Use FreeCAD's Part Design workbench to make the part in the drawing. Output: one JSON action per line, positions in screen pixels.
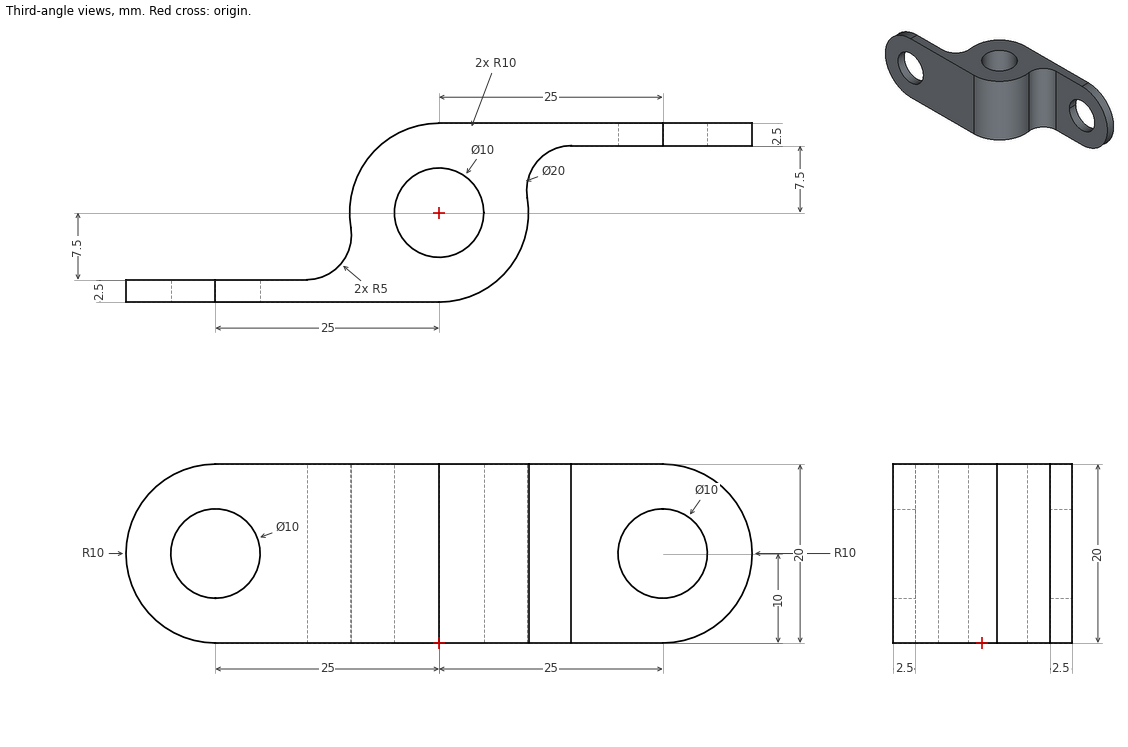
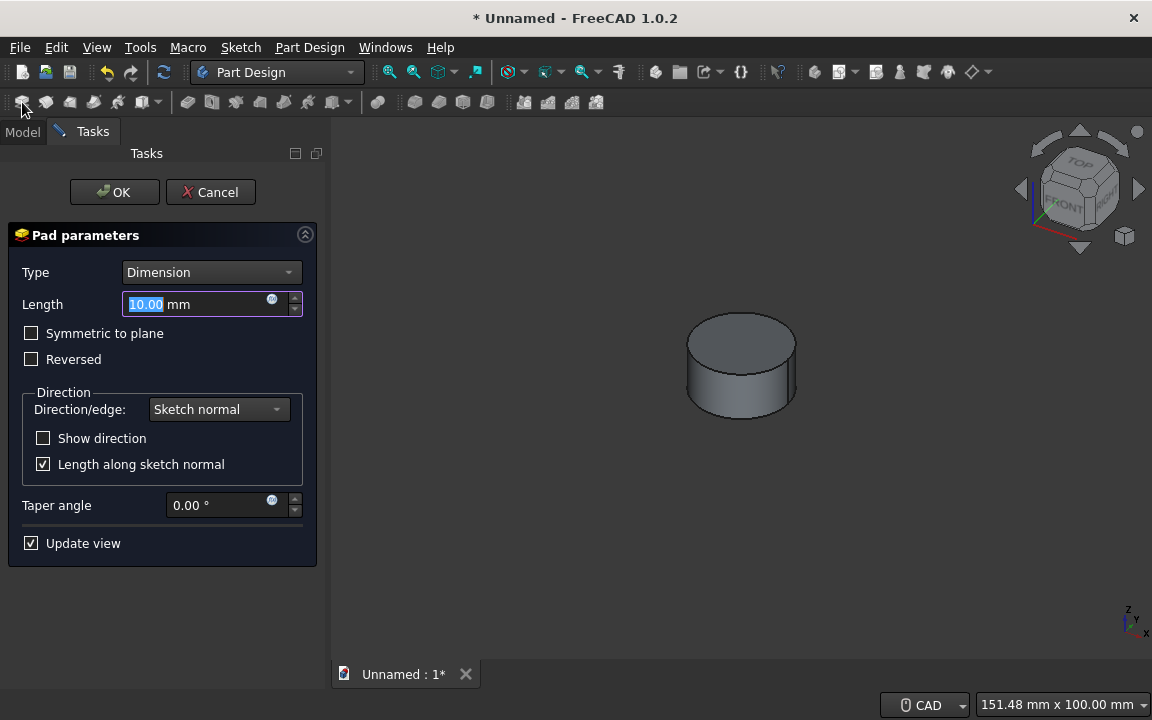
{"action": "type", "text": "20"}
{"action": "key", "text": "Tab"}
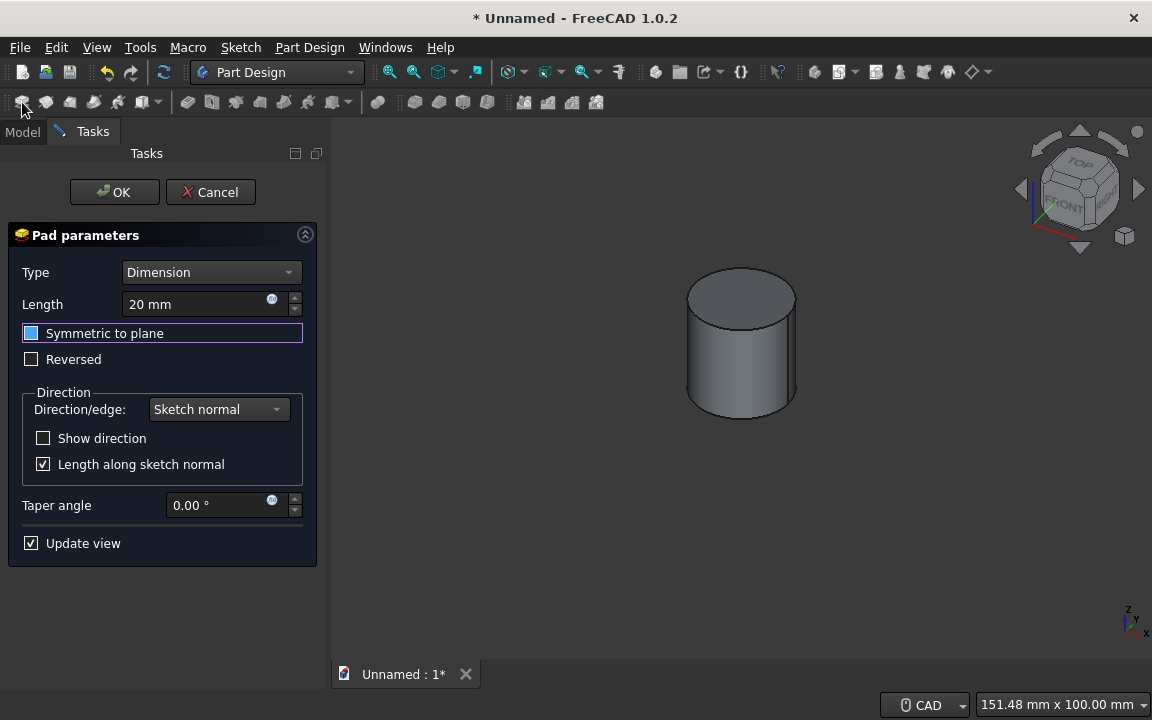
{"action": "left_click", "coordinate": [115, 192]}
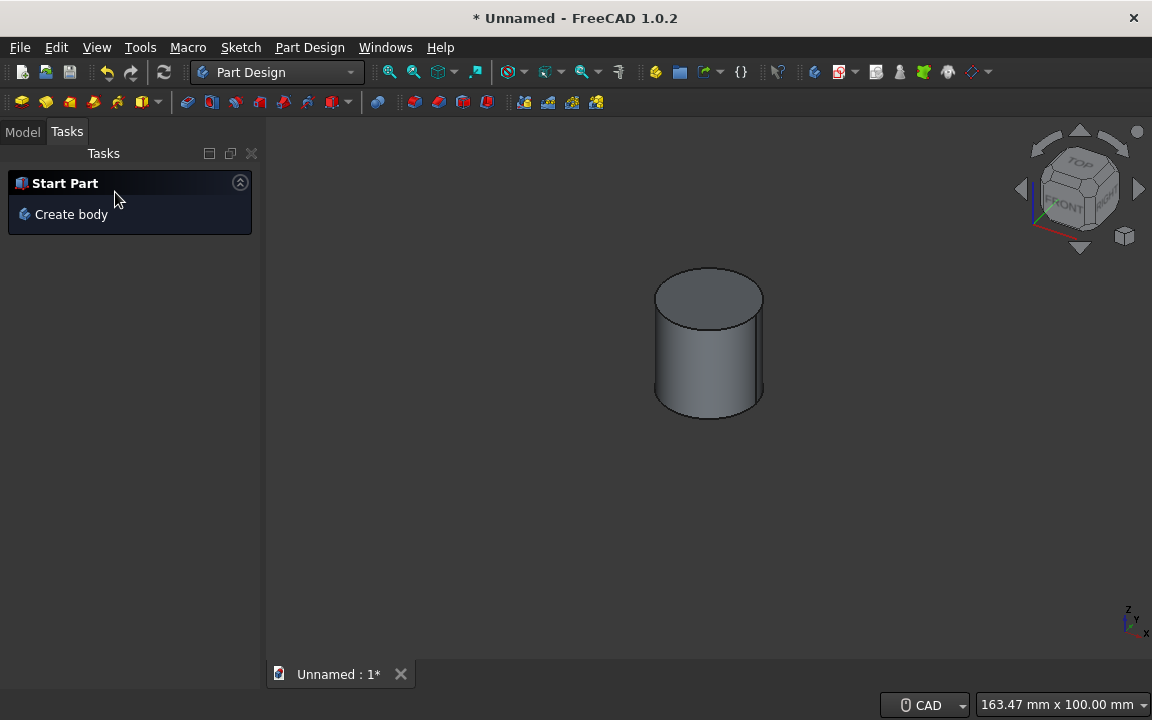
{"action": "left_click", "coordinate": [390, 72]}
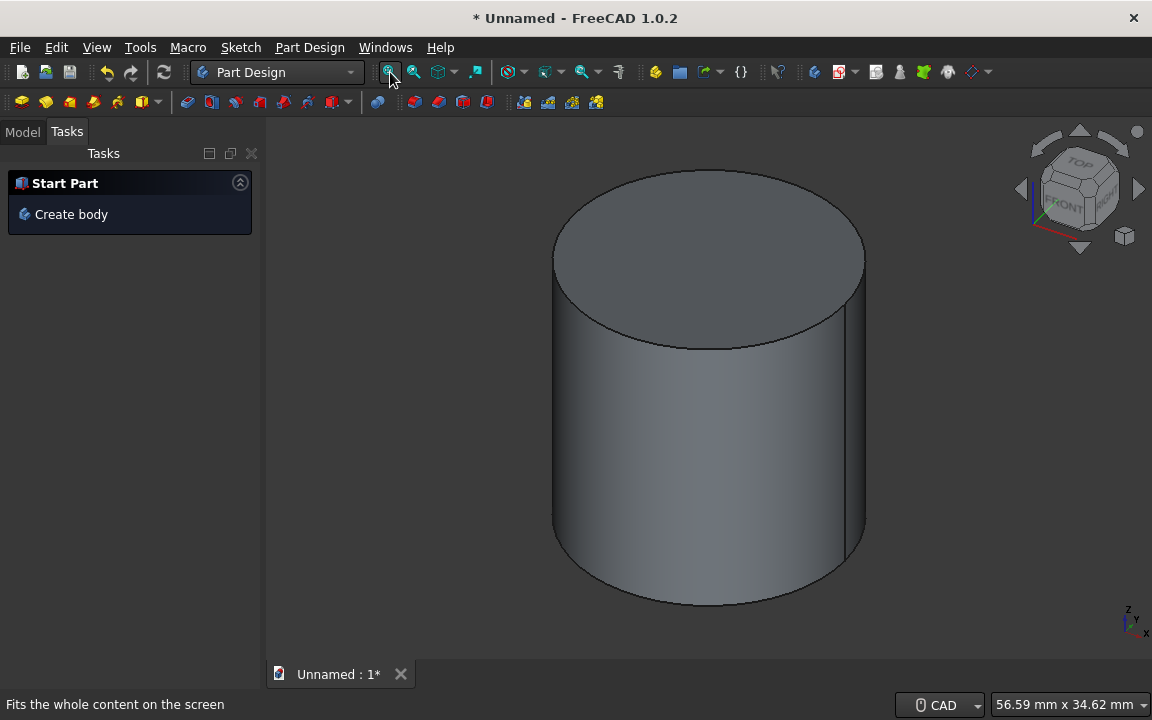
{"action": "key", "text": "5"}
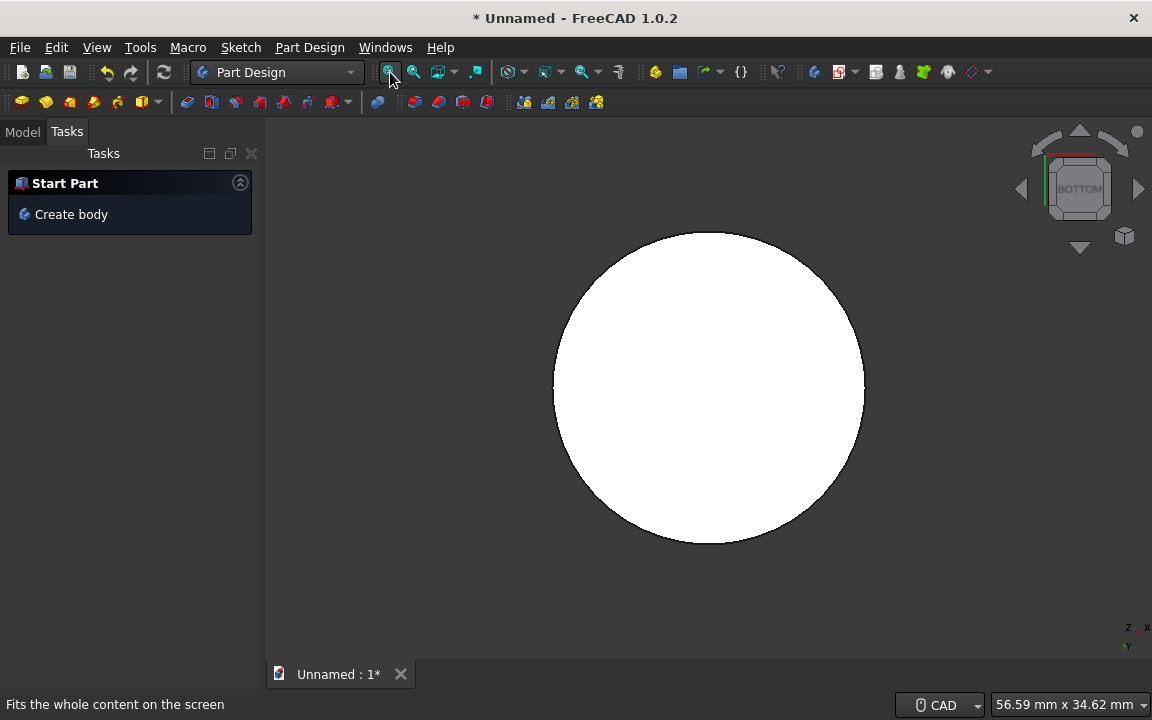
{"action": "left_click", "coordinate": [709, 387]}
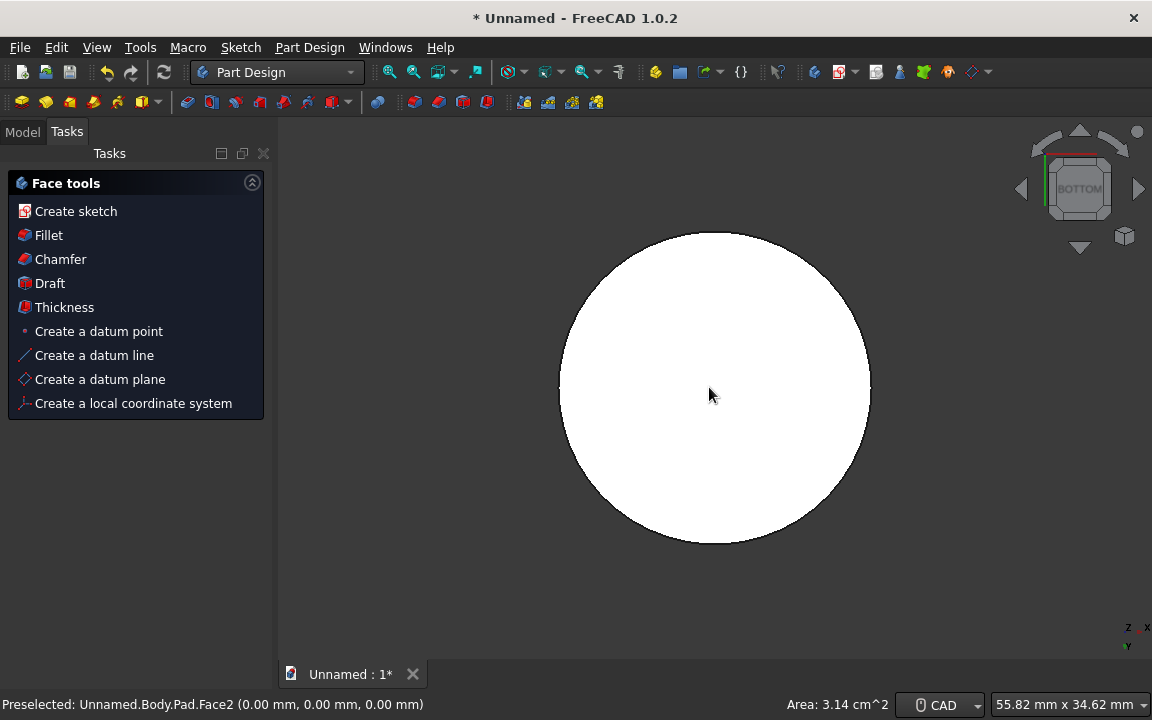
{"action": "left_click", "coordinate": [840, 72]}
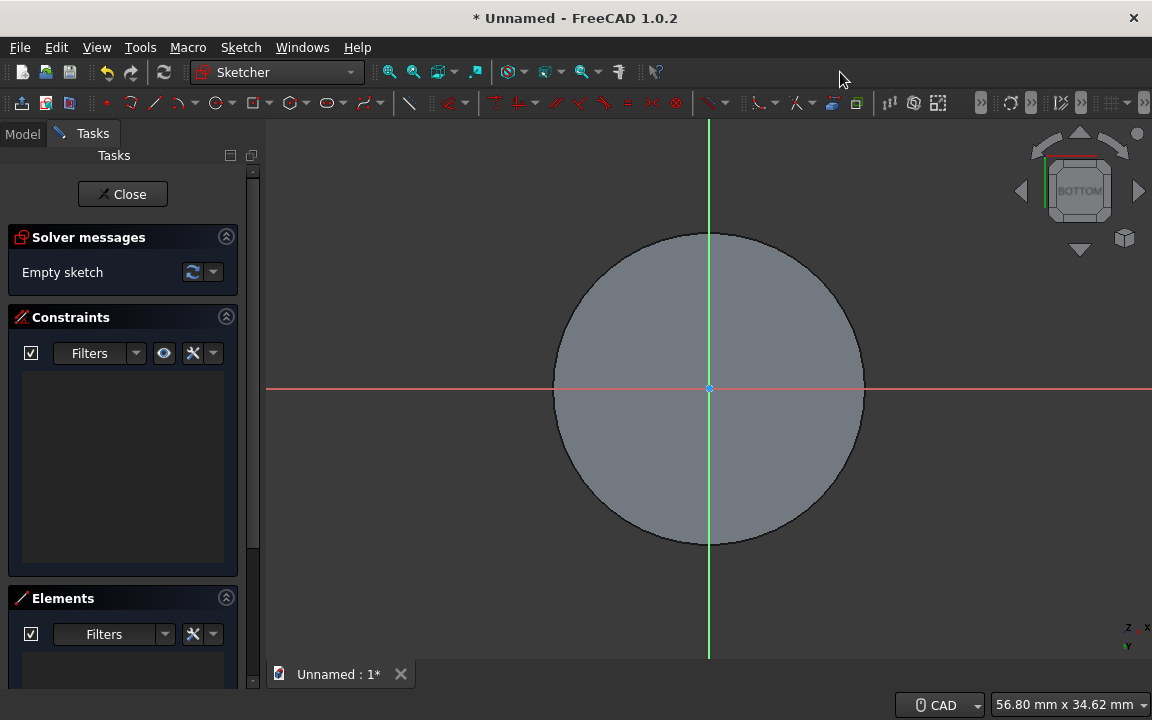
{"action": "scroll", "coordinate": [501, 389], "scroll_direction": "down", "scroll_amount": 2}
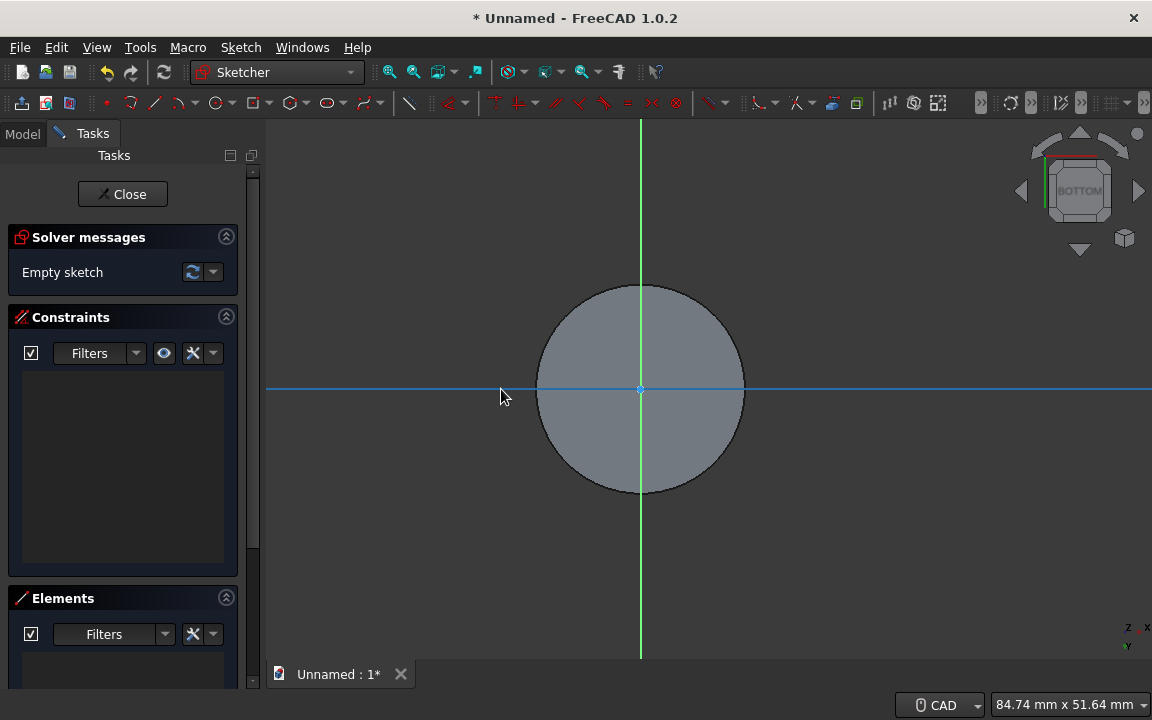
{"action": "left_click", "coordinate": [132, 104]}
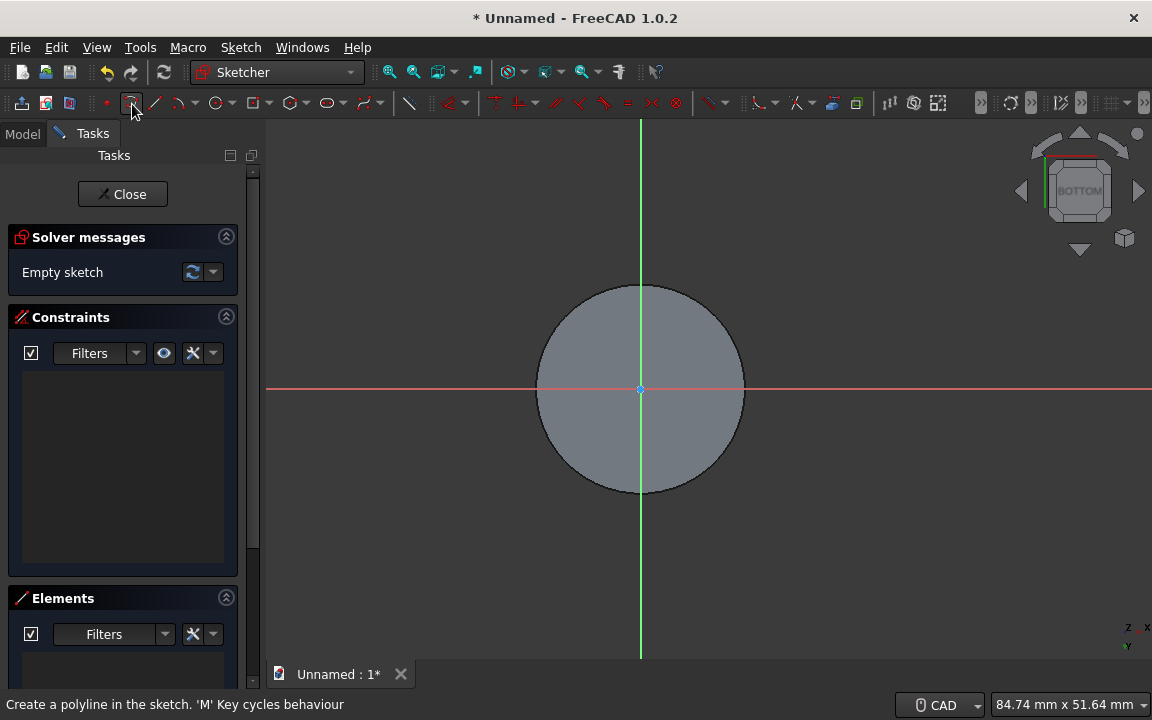
{"action": "left_click", "coordinate": [710, 468]}
{"action": "left_click", "coordinate": [902, 468]}
{"action": "left_click", "coordinate": [902, 494]}
{"action": "left_click", "coordinate": [641, 494]}
{"action": "right_click", "coordinate": [641, 494]}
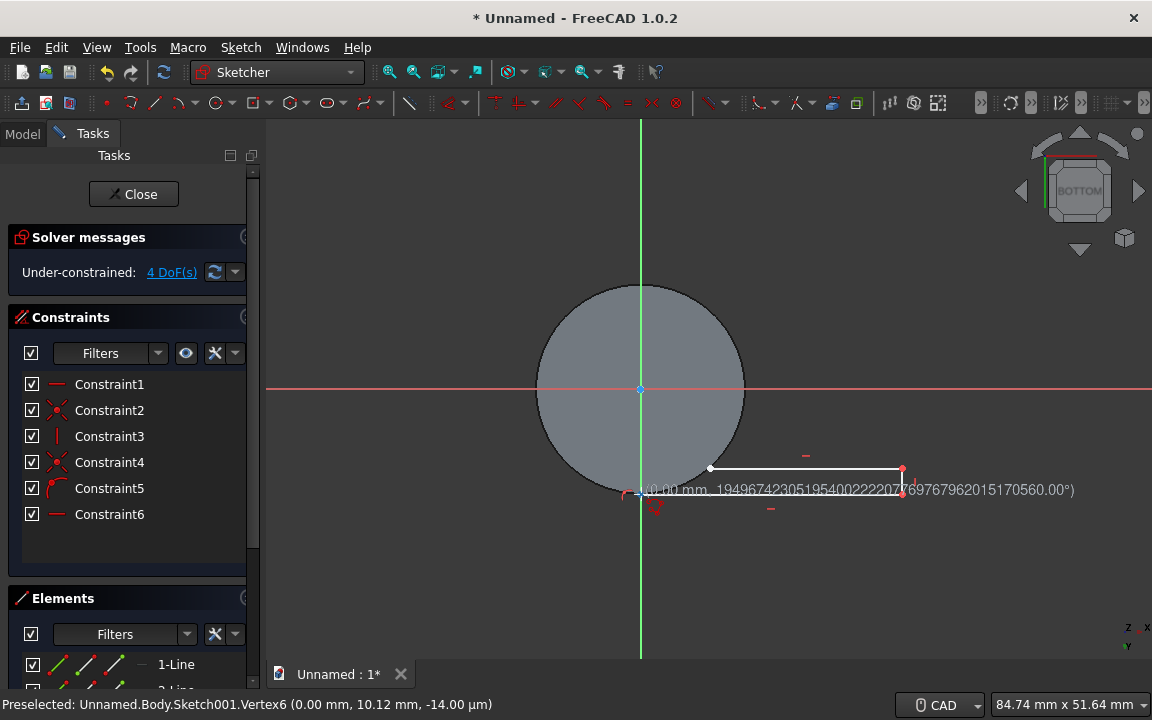
{"action": "key", "text": "g 3 a"}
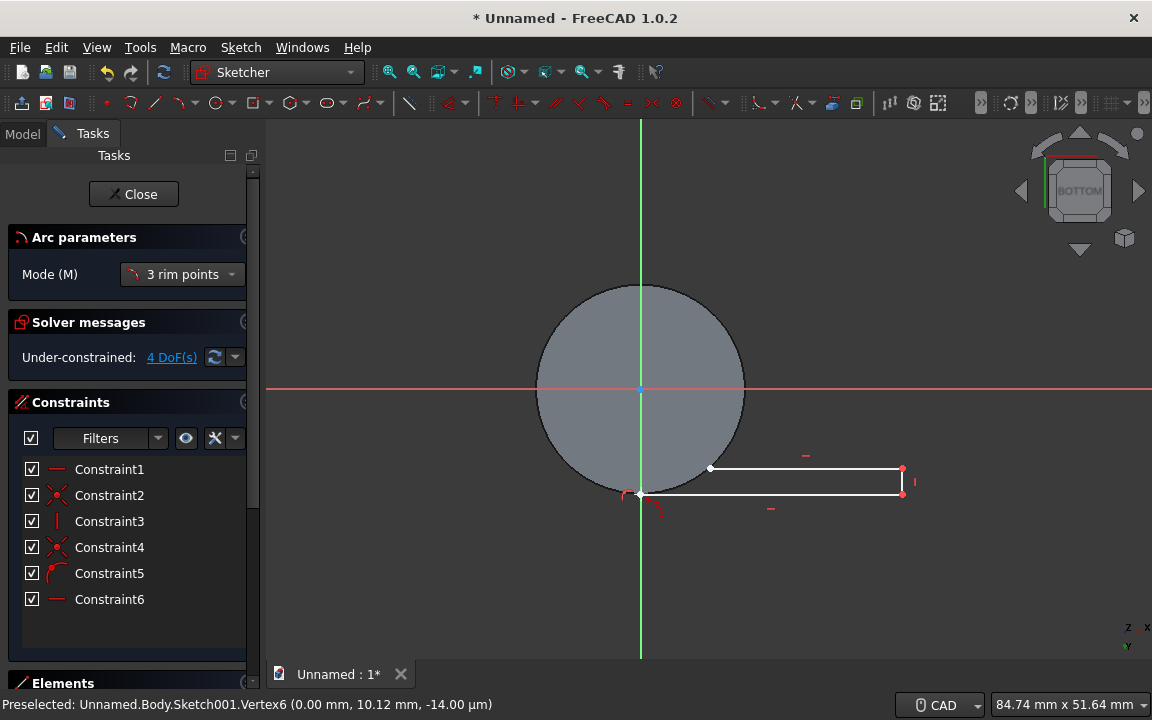
{"action": "left_click", "coordinate": [641, 495]}
{"action": "left_click", "coordinate": [710, 469]}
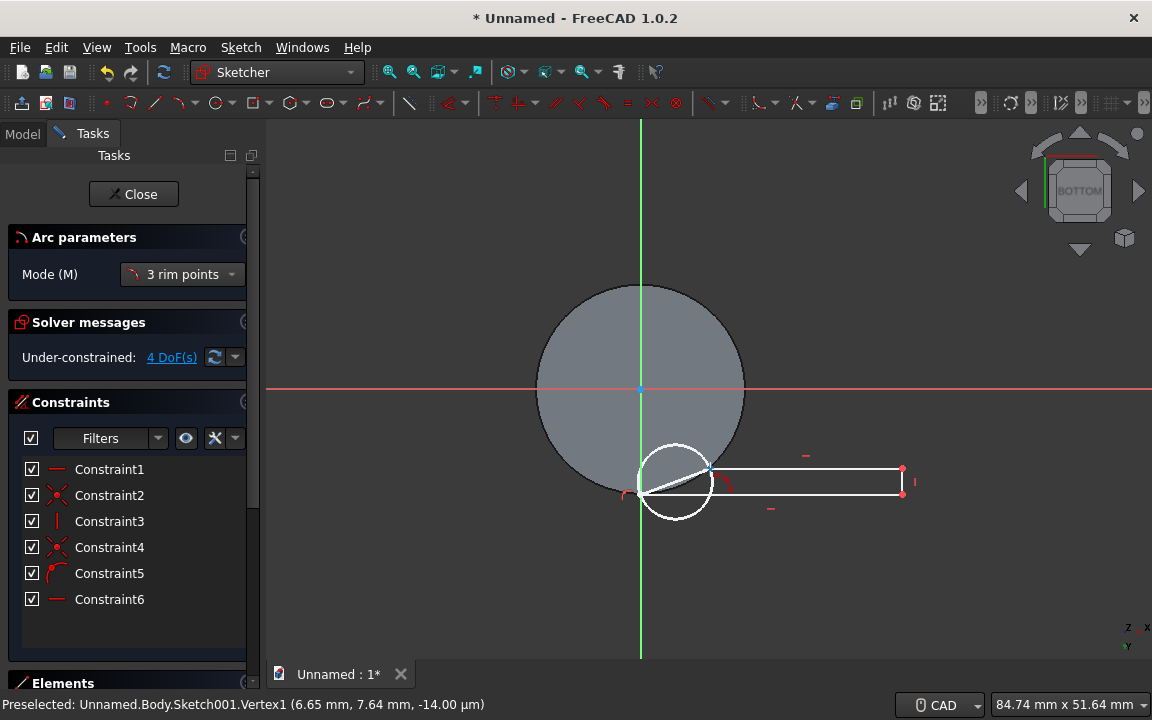
{"action": "scroll", "coordinate": [677, 487], "scroll_direction": "up", "scroll_amount": 5}